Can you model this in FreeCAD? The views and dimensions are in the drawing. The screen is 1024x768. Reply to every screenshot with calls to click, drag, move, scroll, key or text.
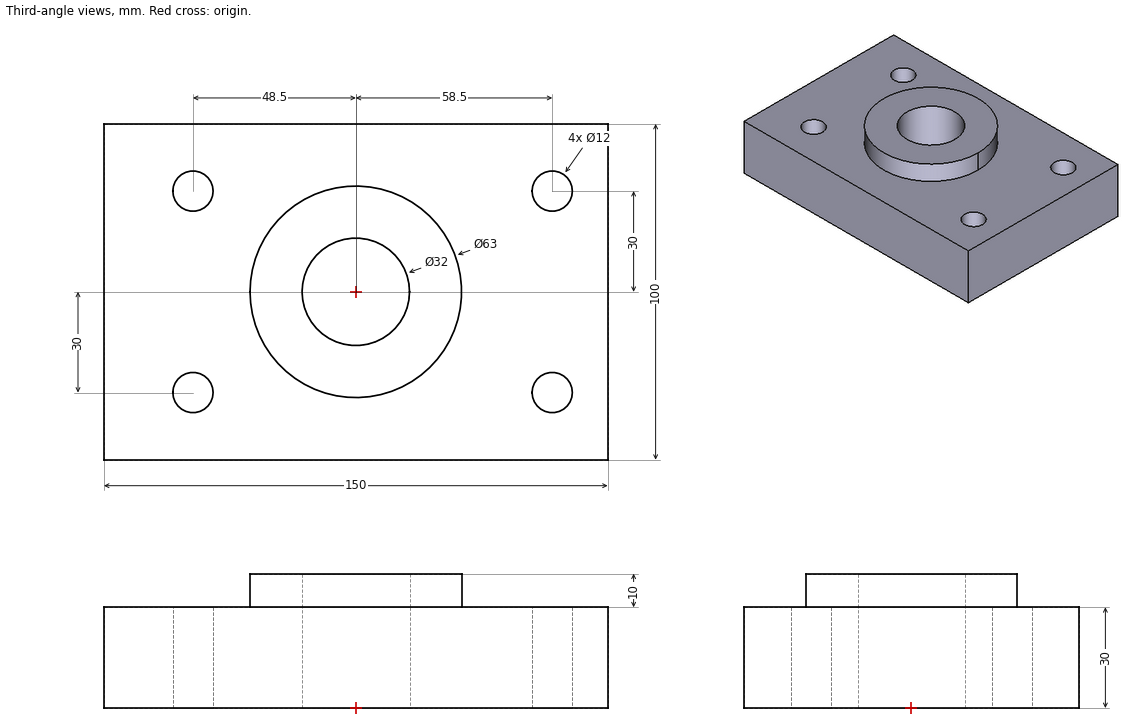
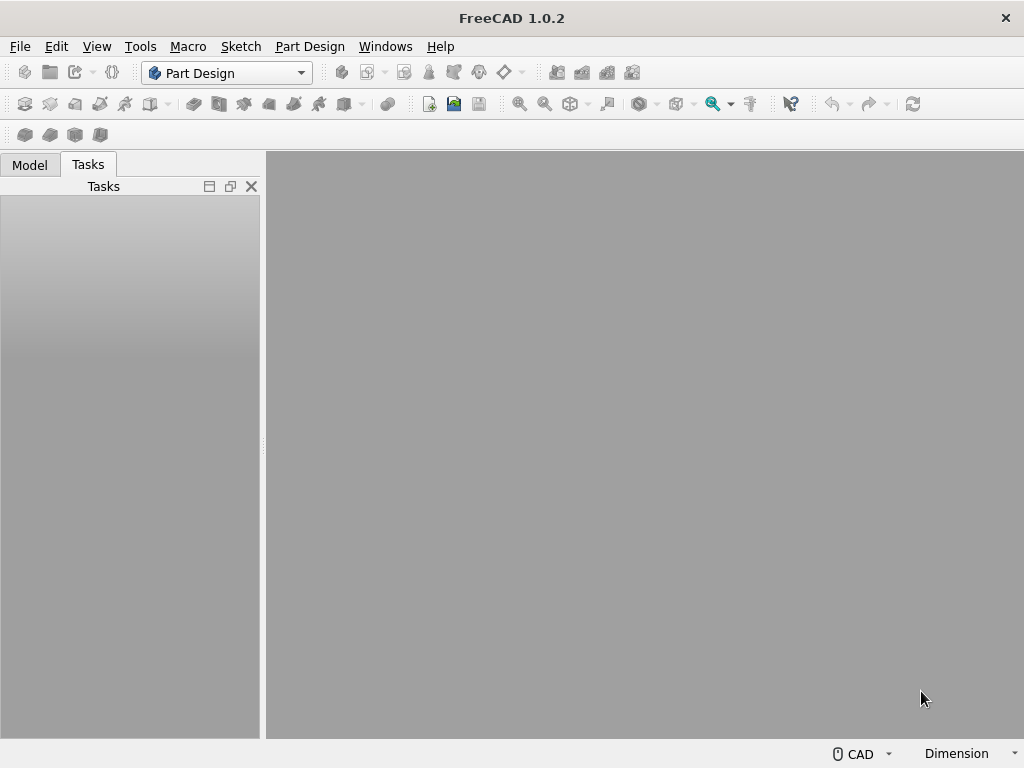
click(429, 104)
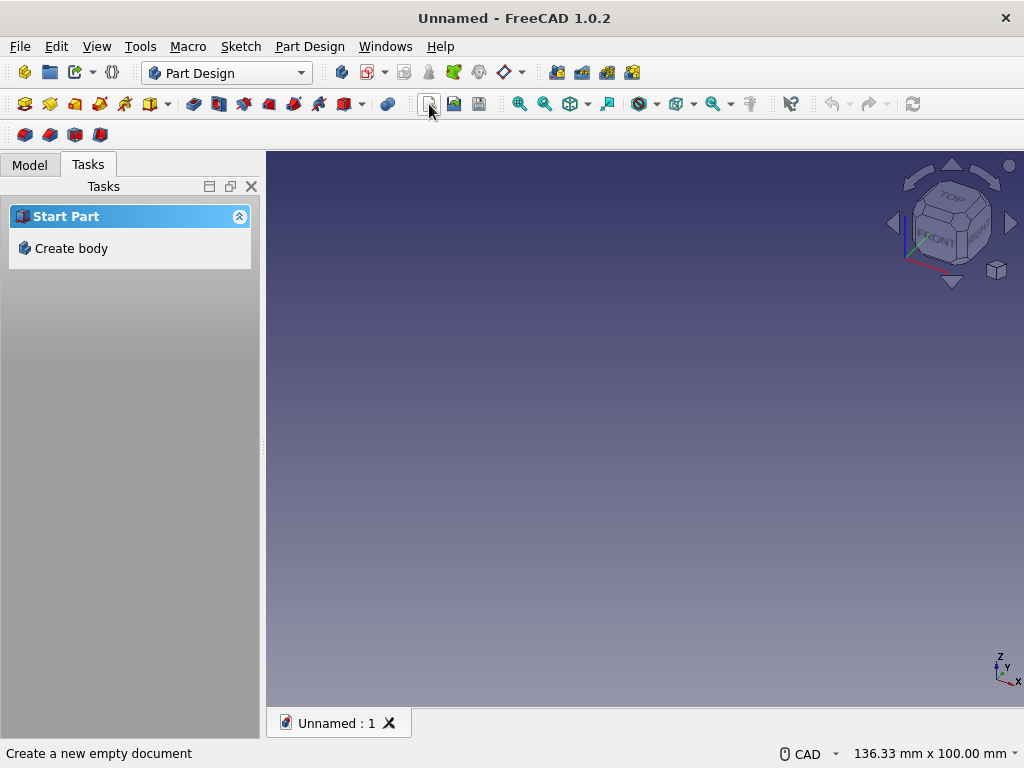
click(366, 72)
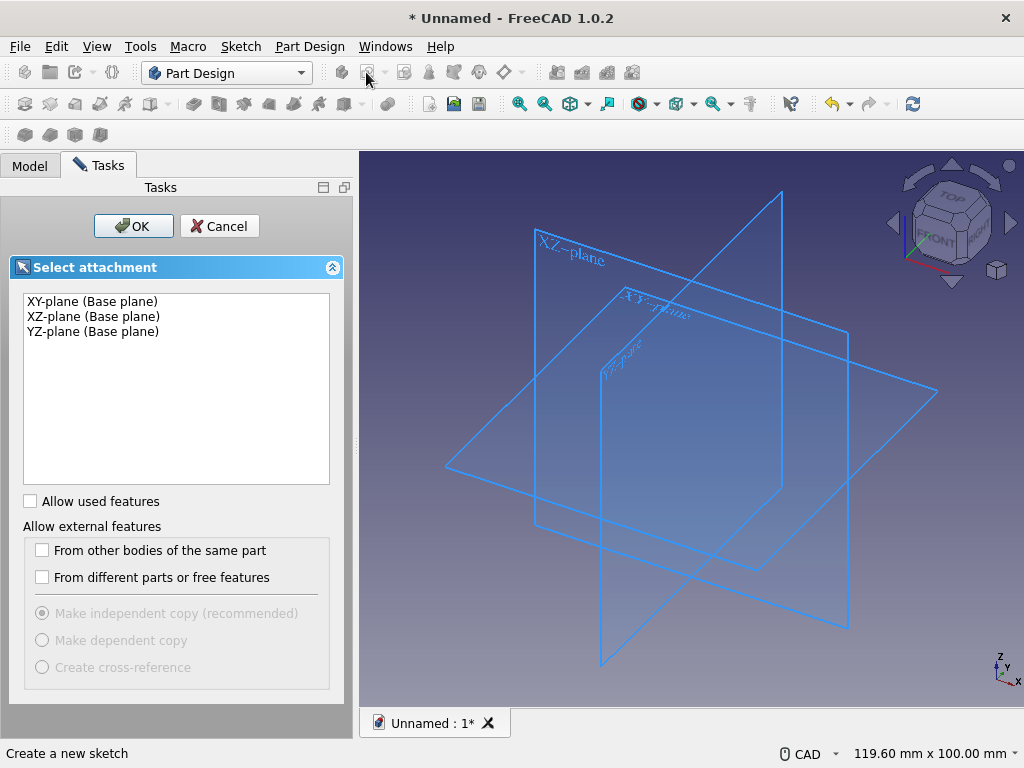
click(84, 302)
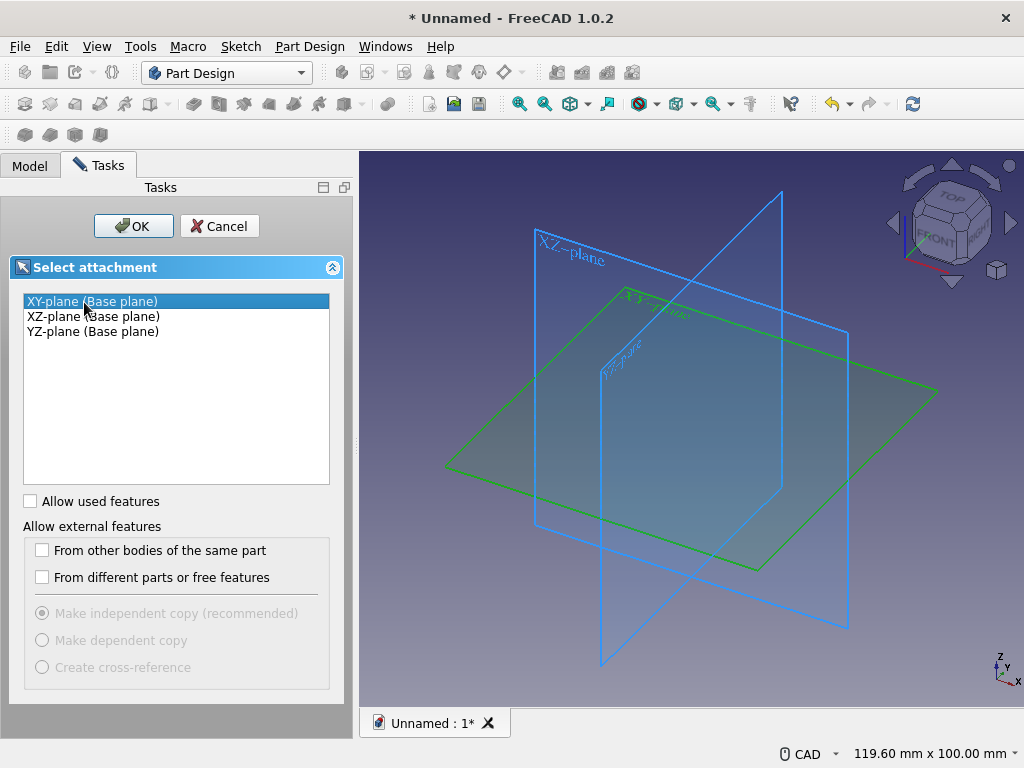
click(134, 226)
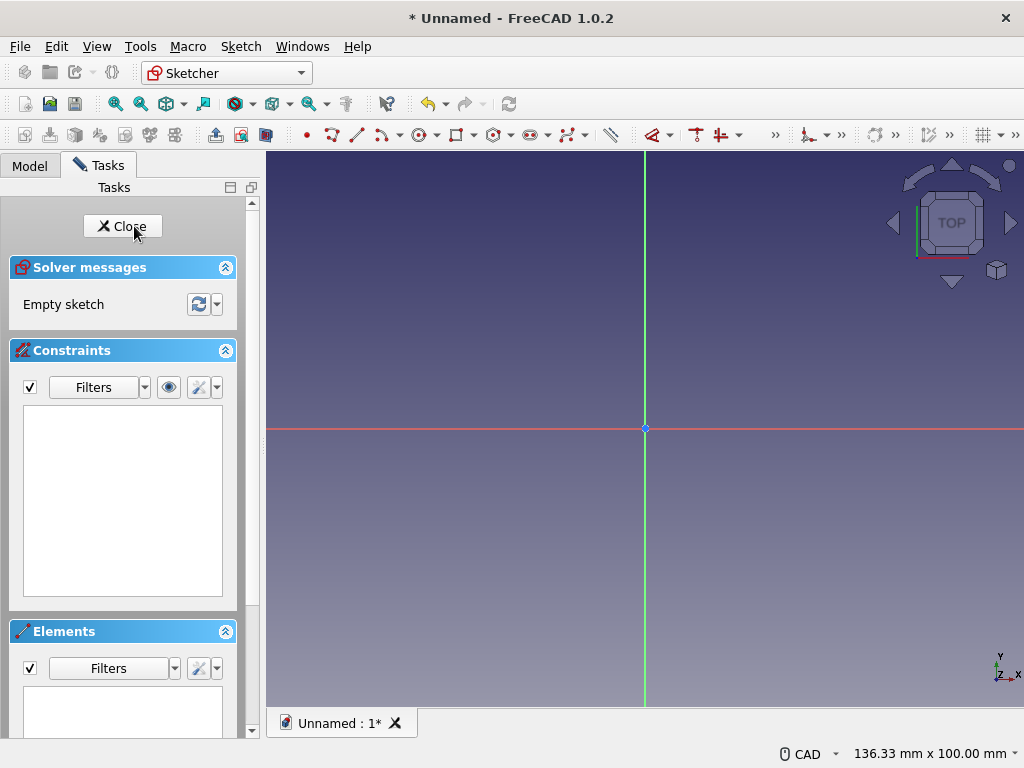
scroll(521, 429, down, 4)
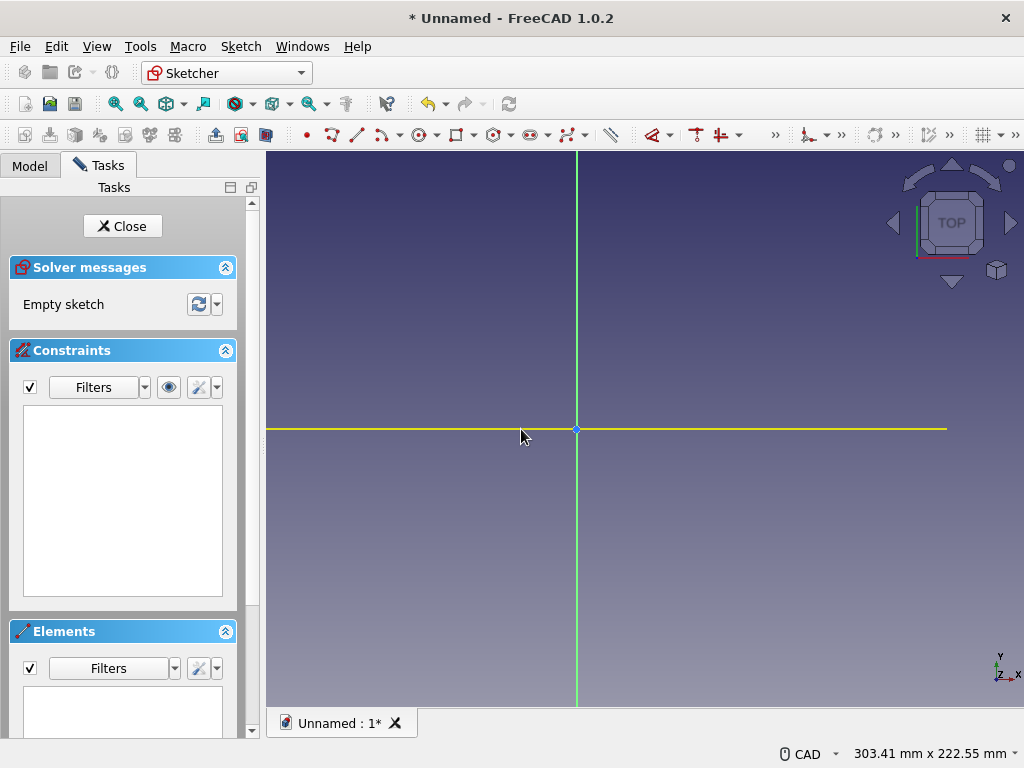
key(g)
key(v)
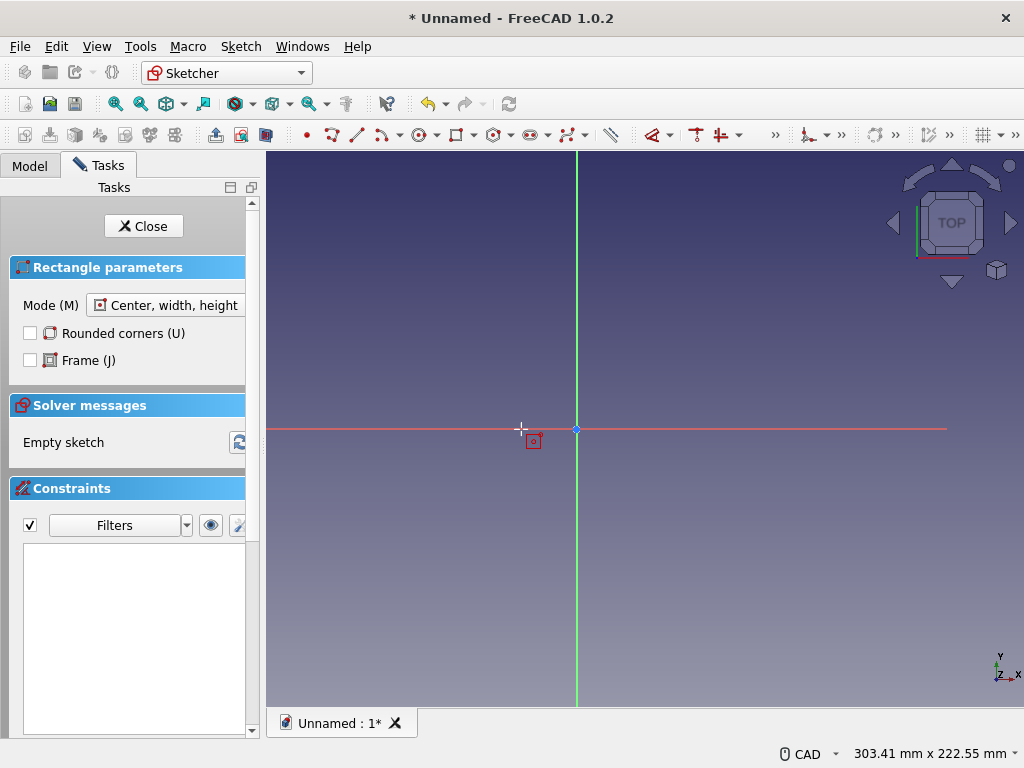
click(577, 429)
move(764, 304)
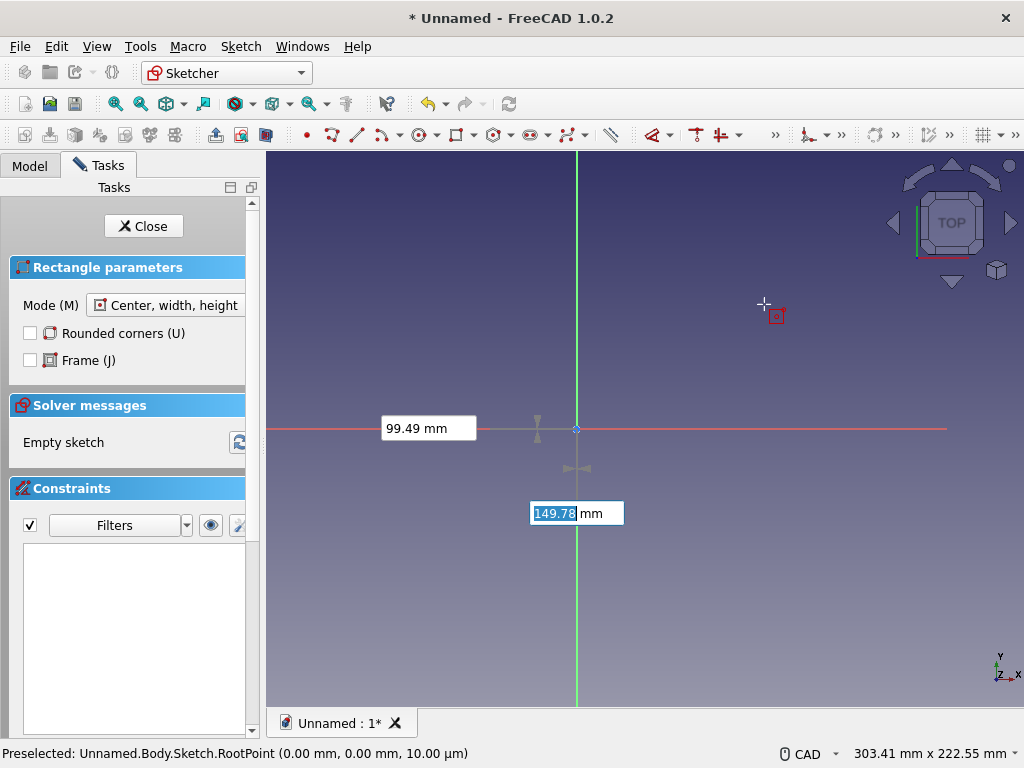
text(150)
key(Tab)
text(100)
key(Return)
key(Escape)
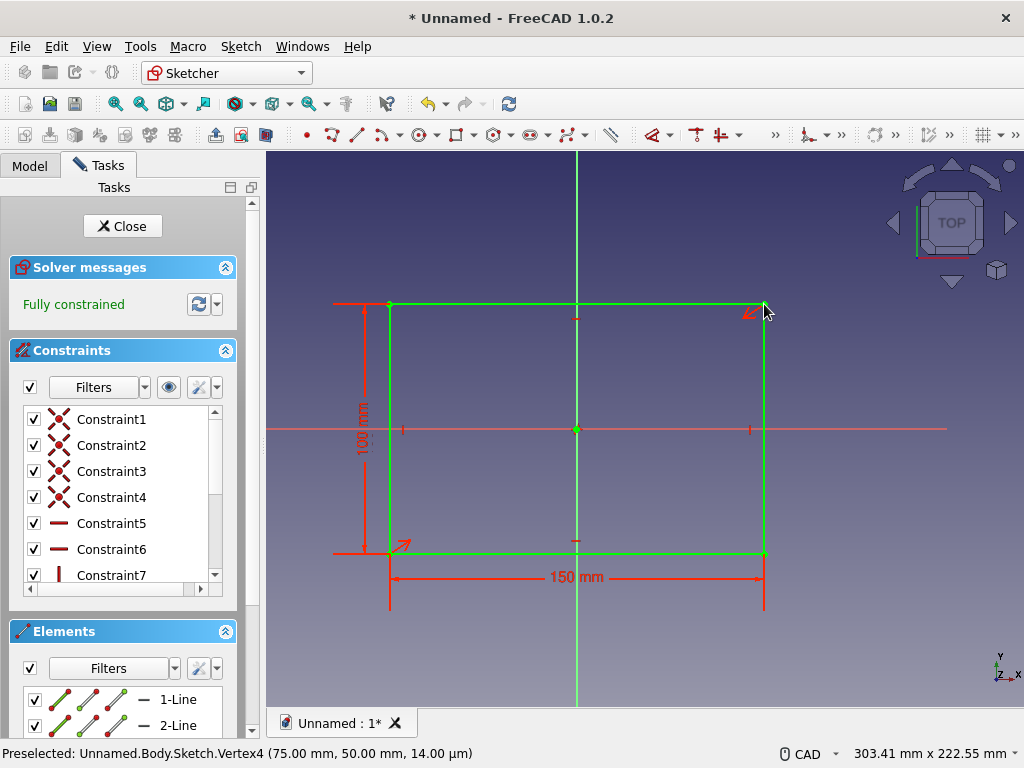
click(123, 226)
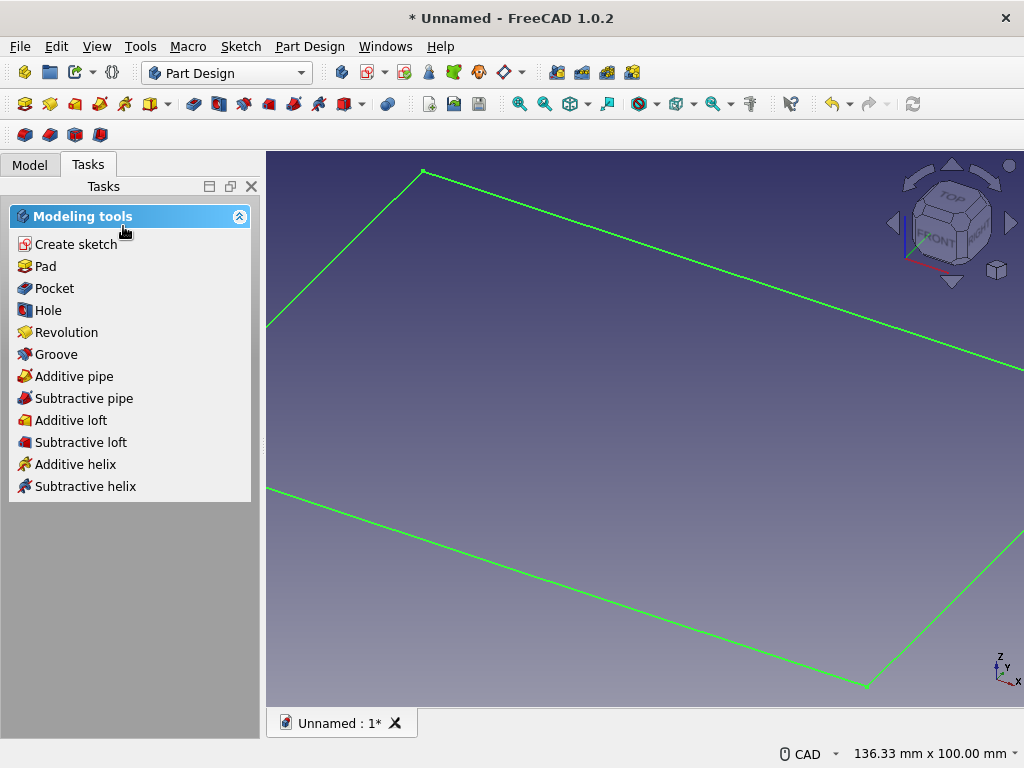
click(25, 104)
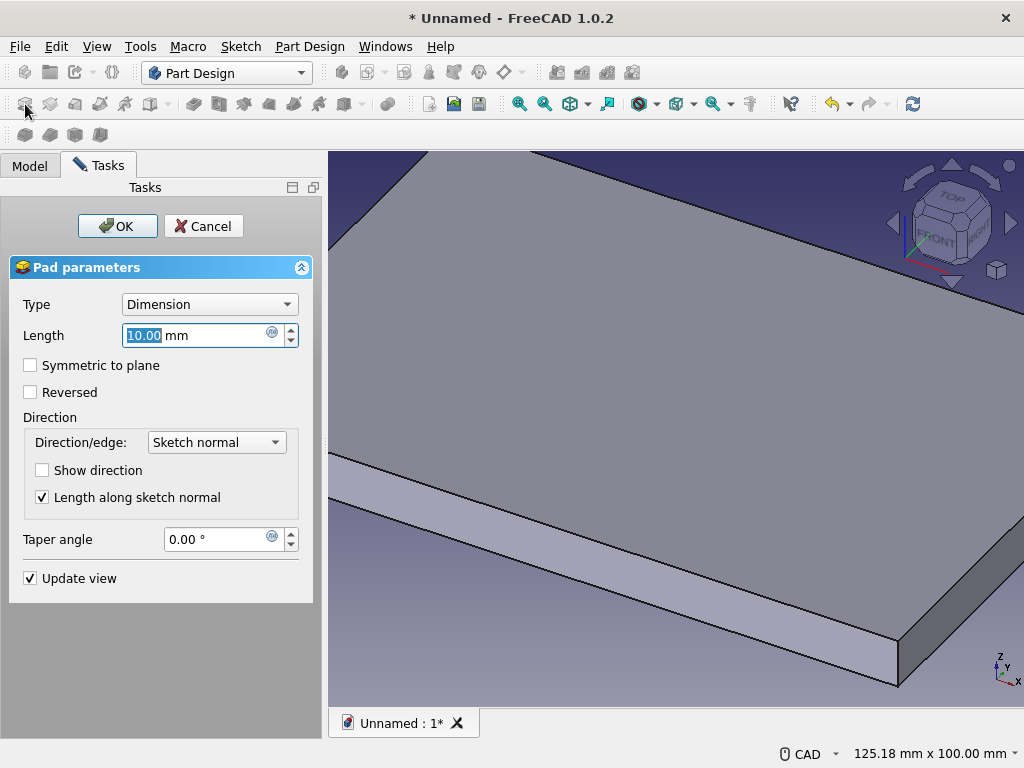
text(30)
key(Tab)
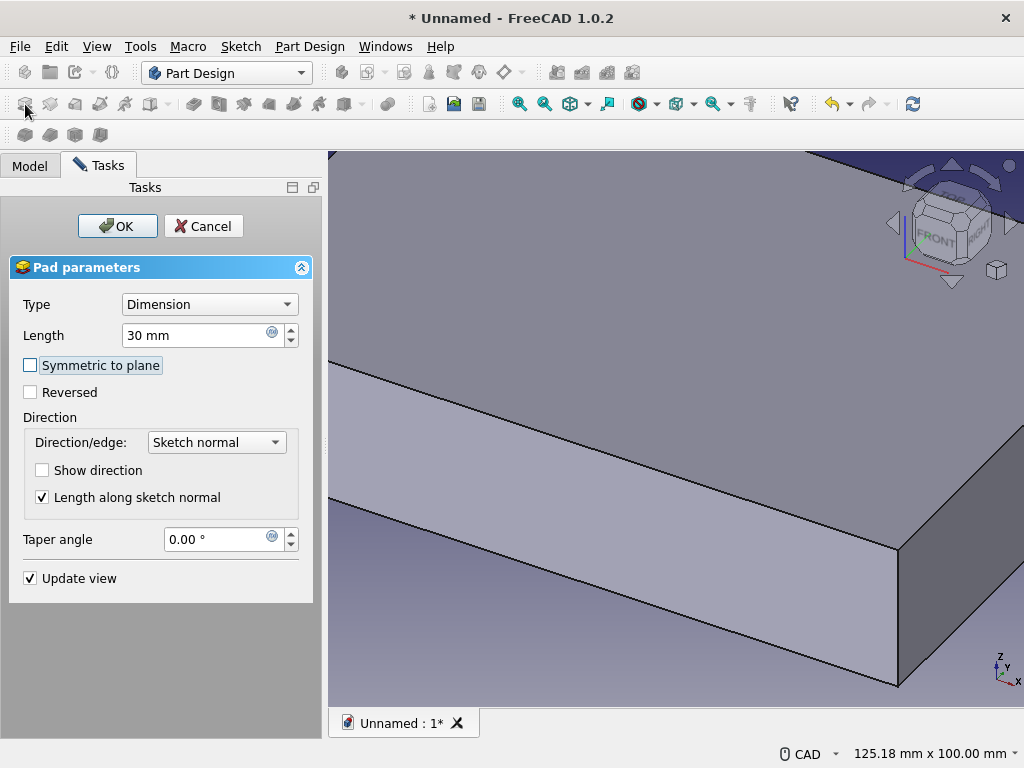
click(118, 226)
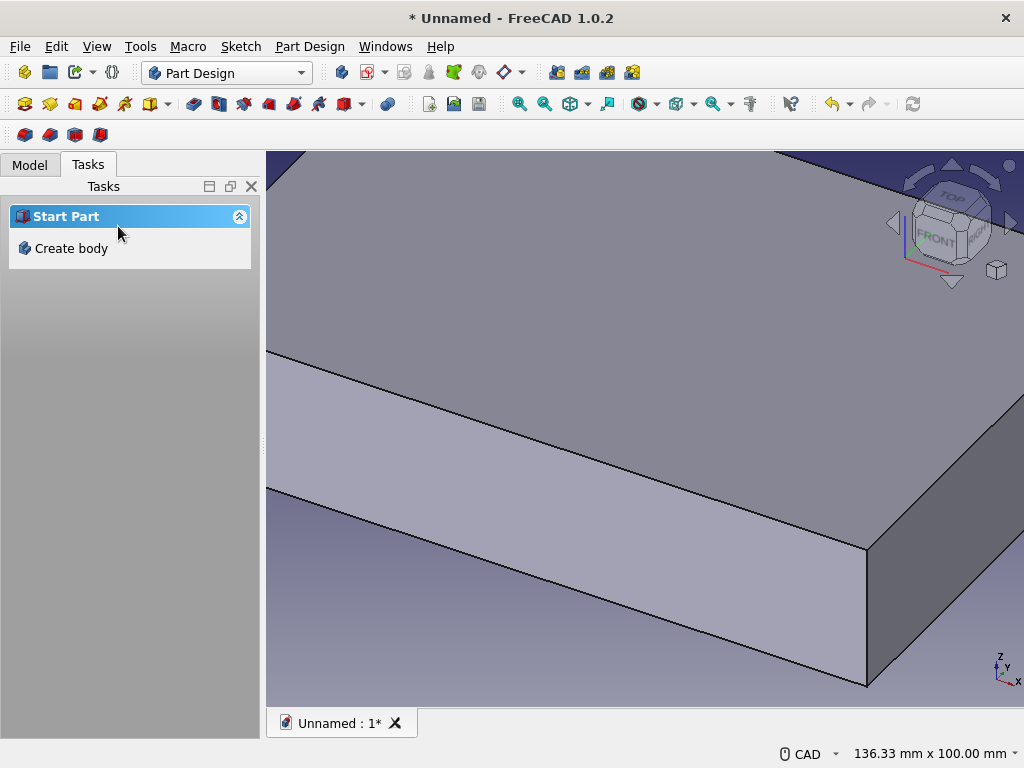
key(v)
key(f)